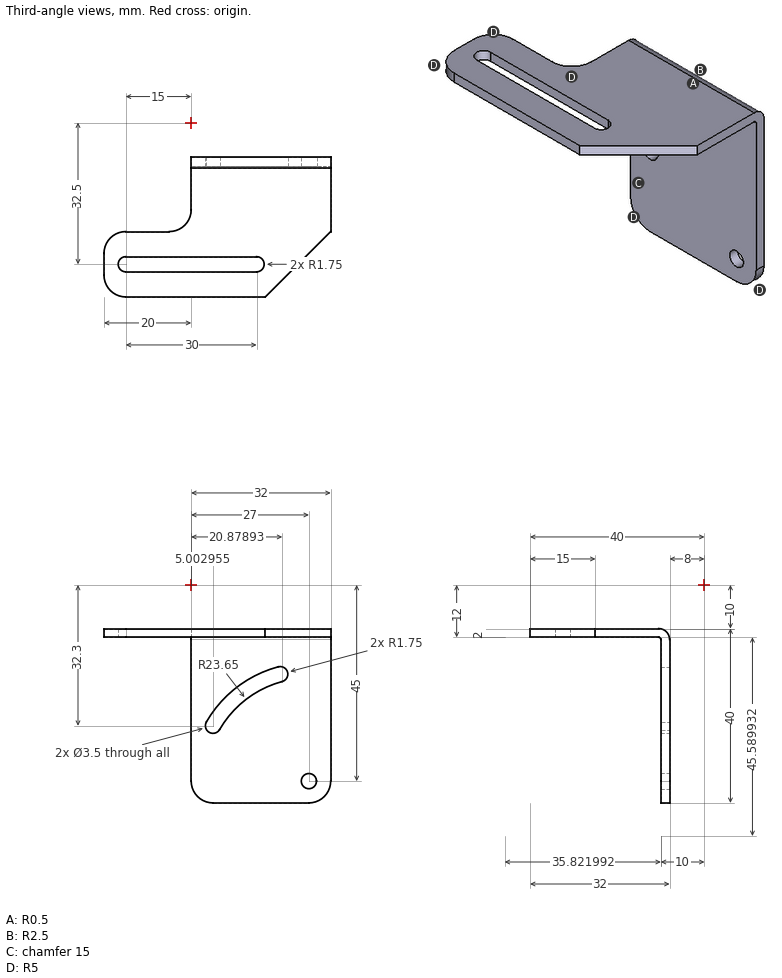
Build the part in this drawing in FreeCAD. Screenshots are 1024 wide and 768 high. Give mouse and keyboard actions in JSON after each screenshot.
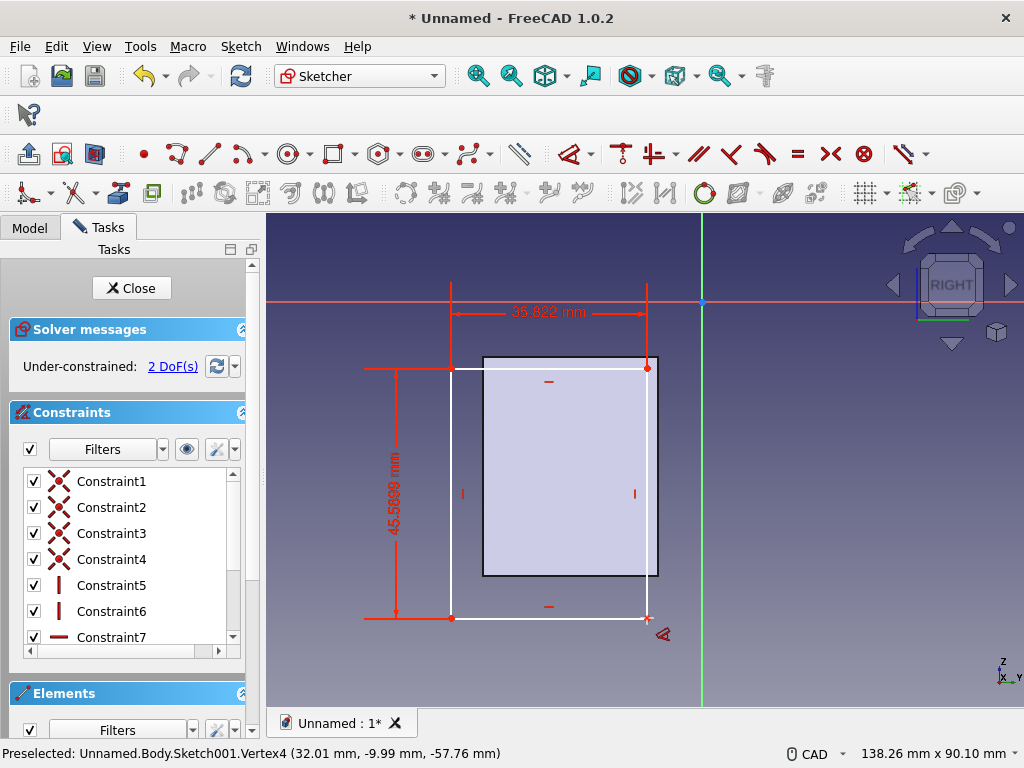
{"action": "left_click", "coordinate": [451, 369]}
{"action": "left_click", "coordinate": [736, 336]}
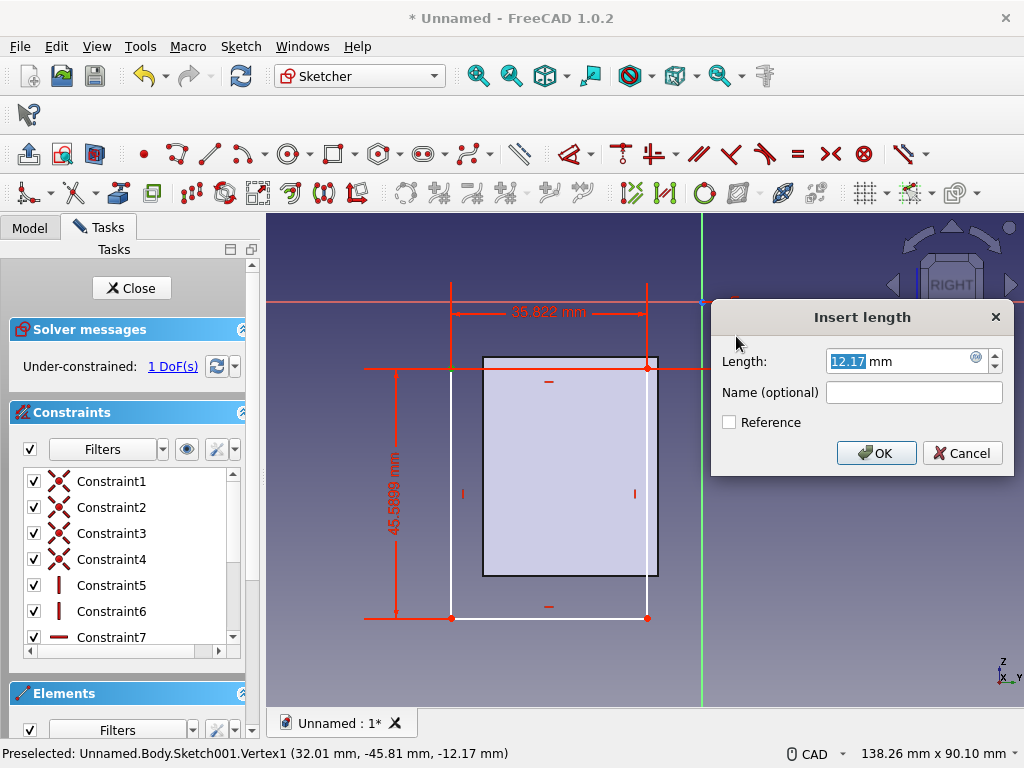
{"action": "type", "text": "12"}
{"action": "key", "text": "Return"}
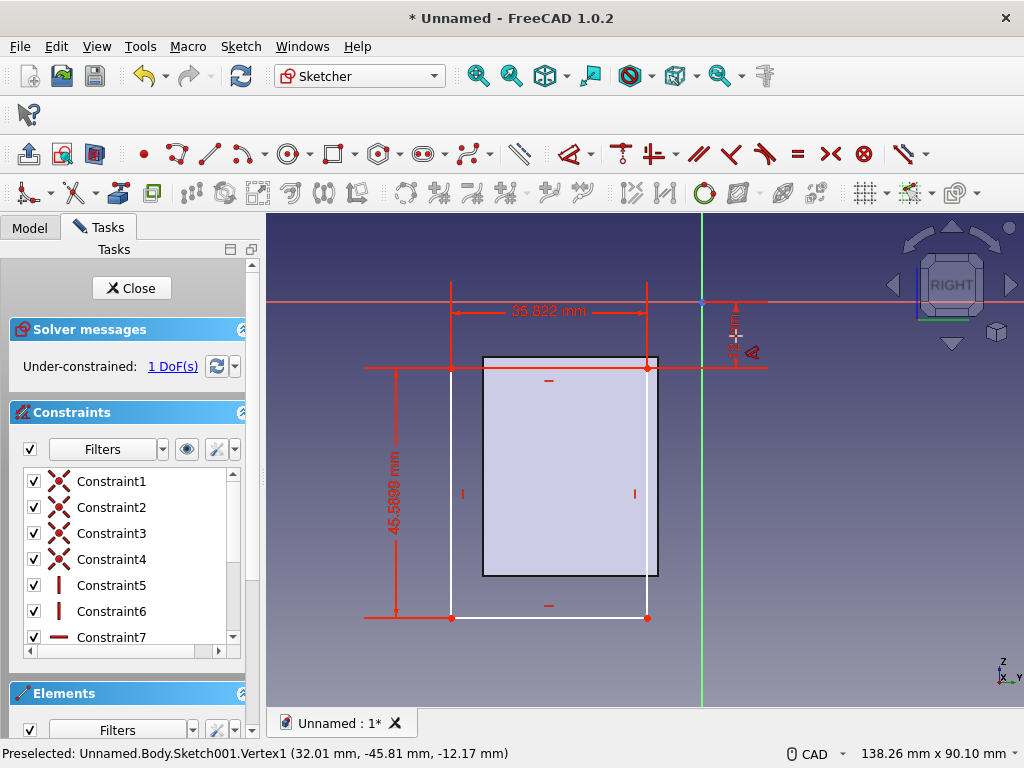
{"action": "left_click", "coordinate": [647, 618]}
{"action": "left_click", "coordinate": [675, 268]}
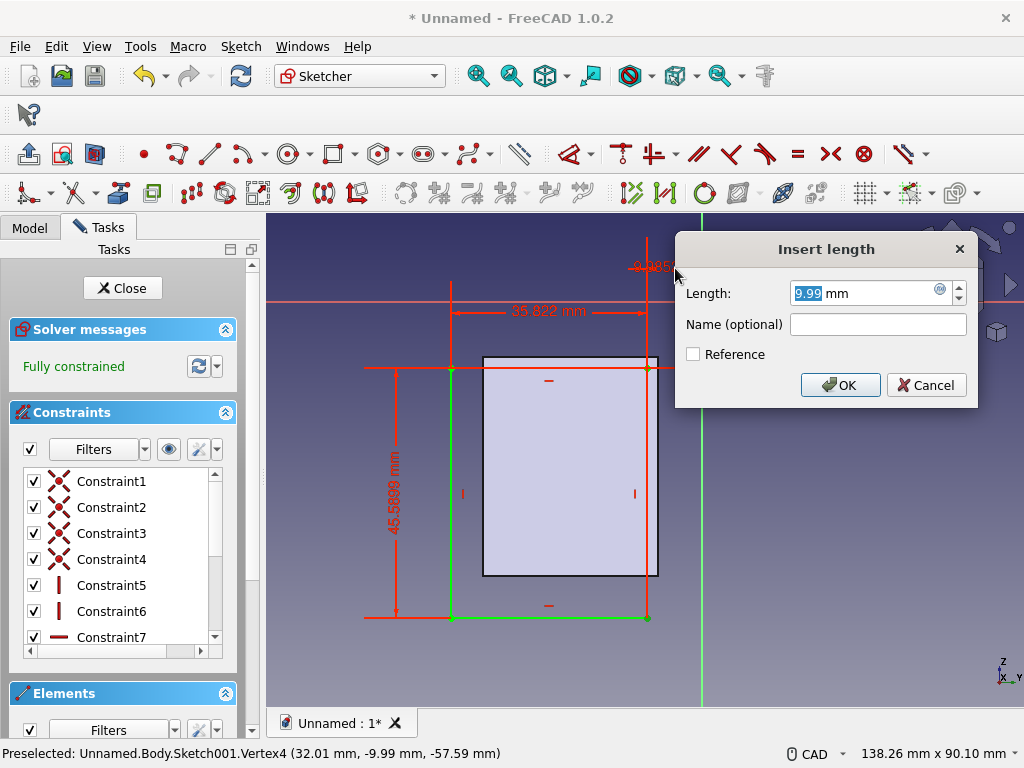
{"action": "type", "text": "10"}
{"action": "key", "text": "Return"}
{"action": "key", "text": "Escape"}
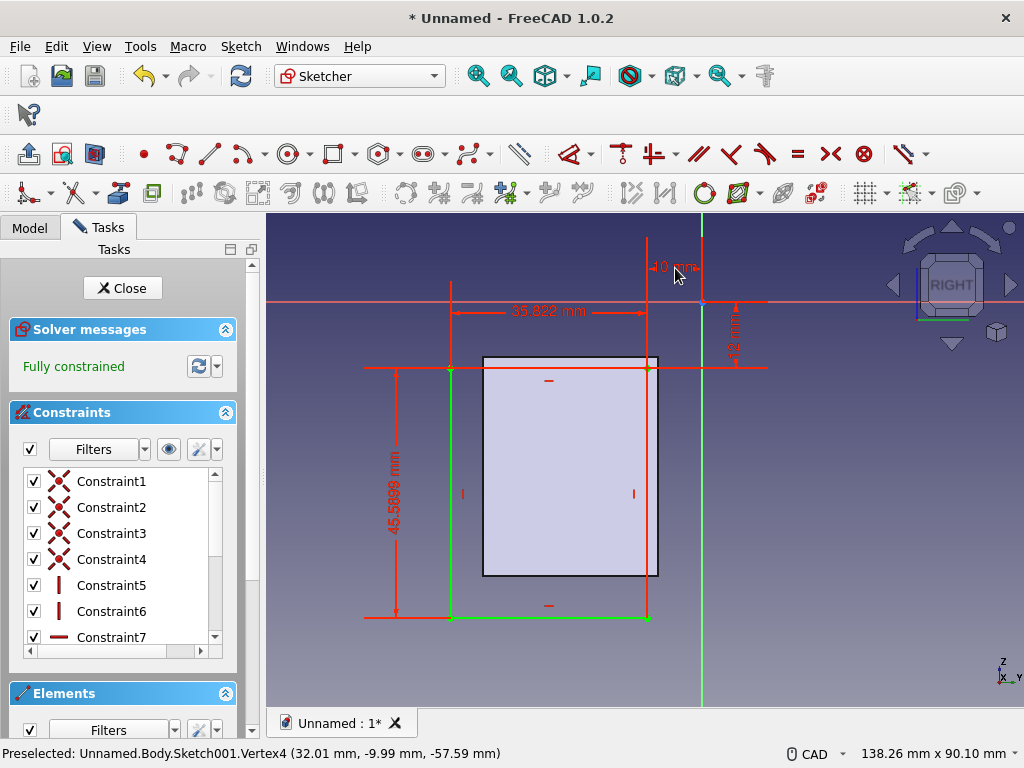
{"action": "left_click", "coordinate": [123, 288]}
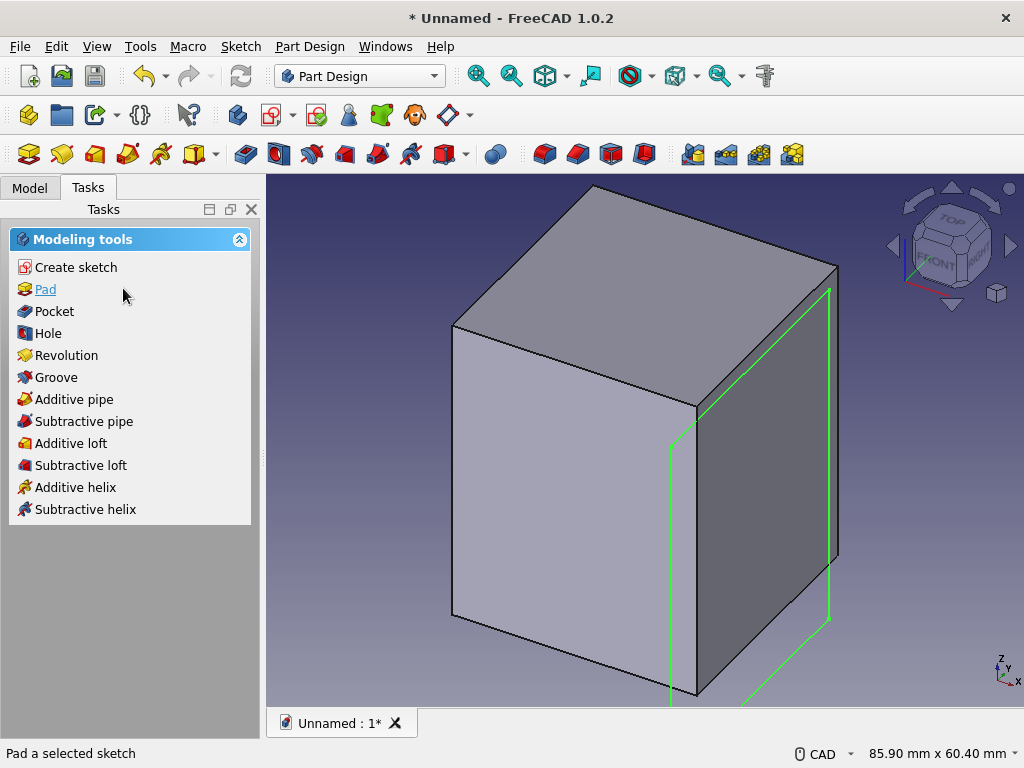
{"action": "left_click", "coordinate": [246, 154]}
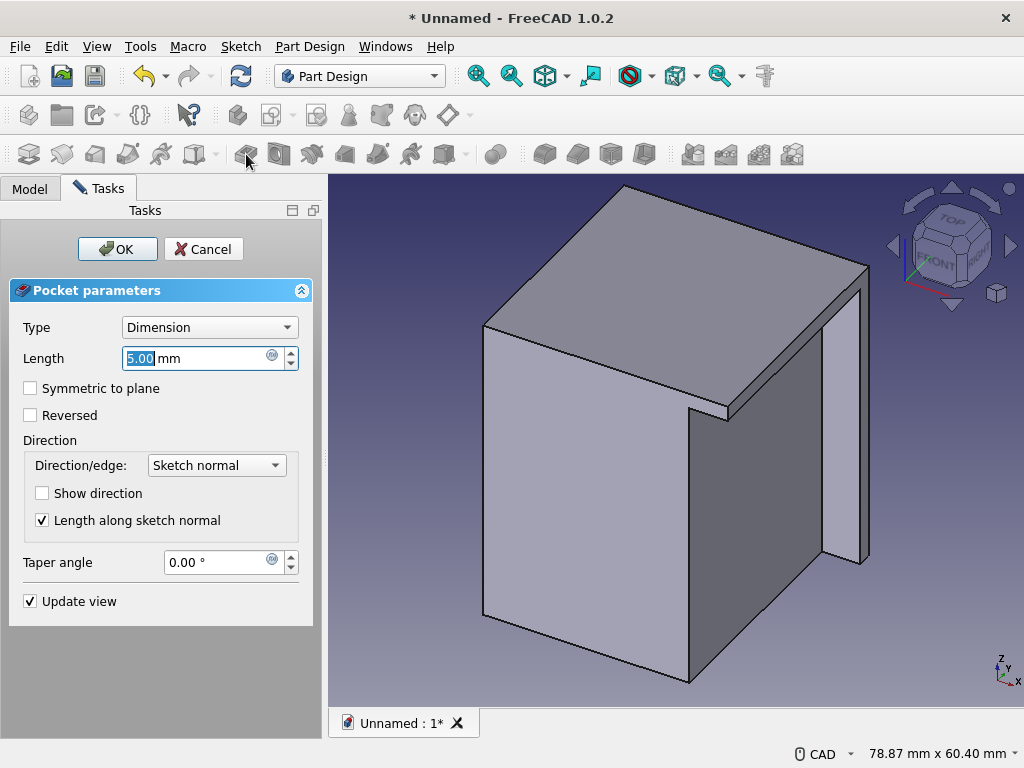
{"action": "left_click", "coordinate": [210, 328]}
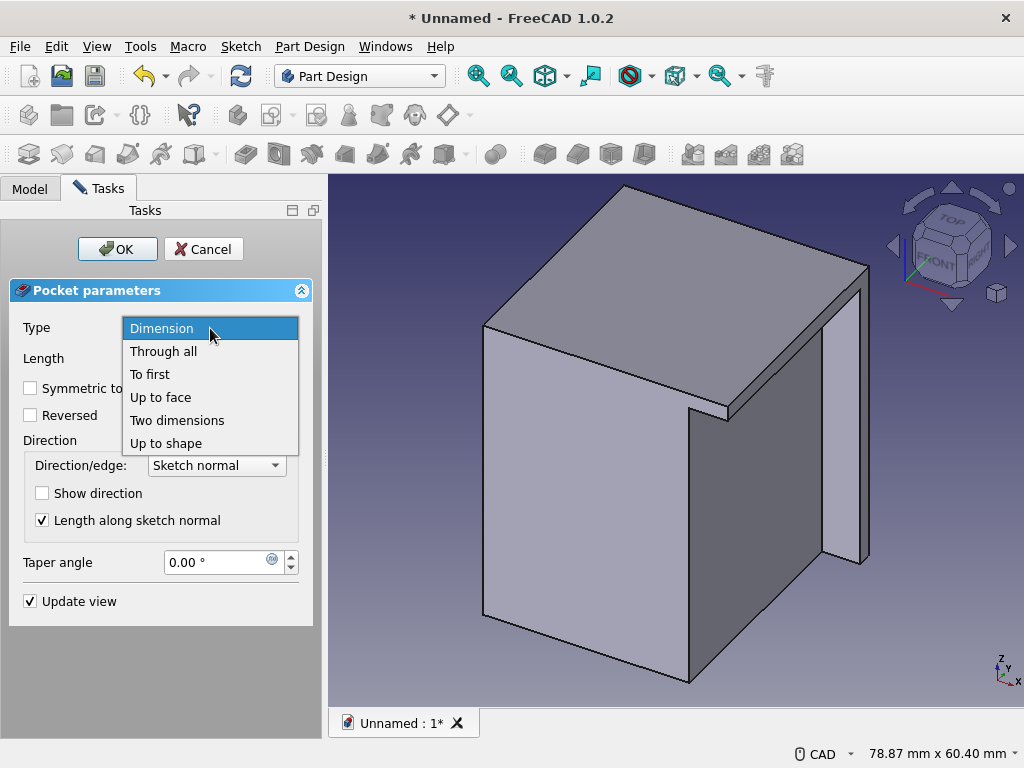
{"action": "left_click", "coordinate": [208, 352]}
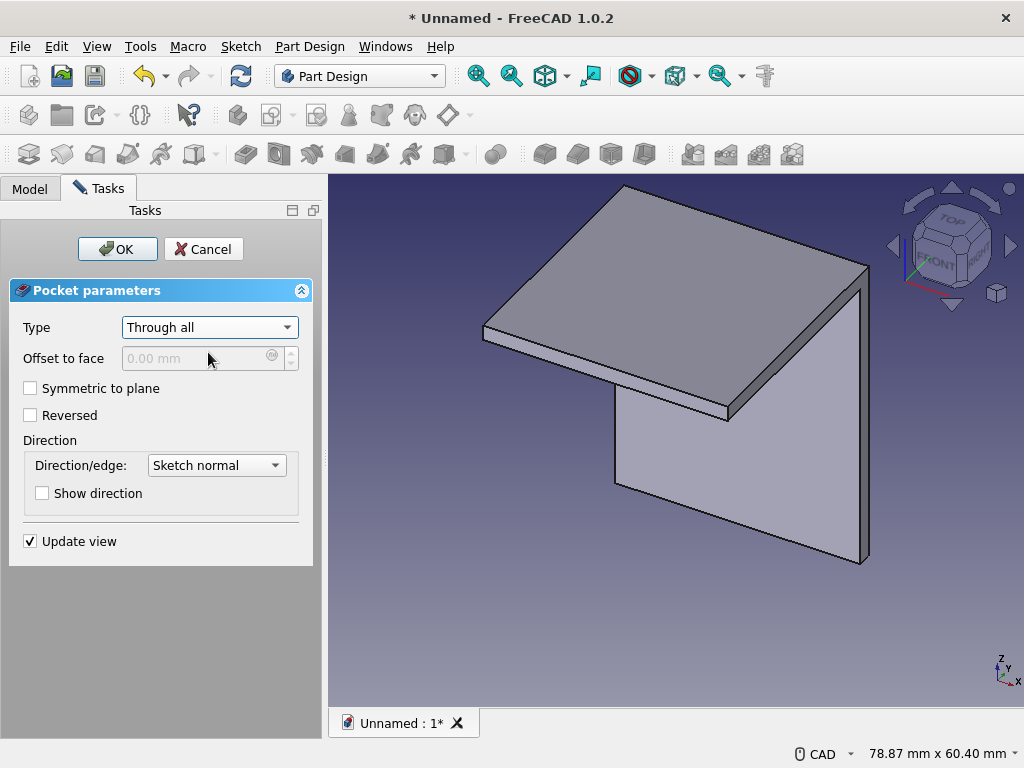
{"action": "left_click", "coordinate": [118, 249]}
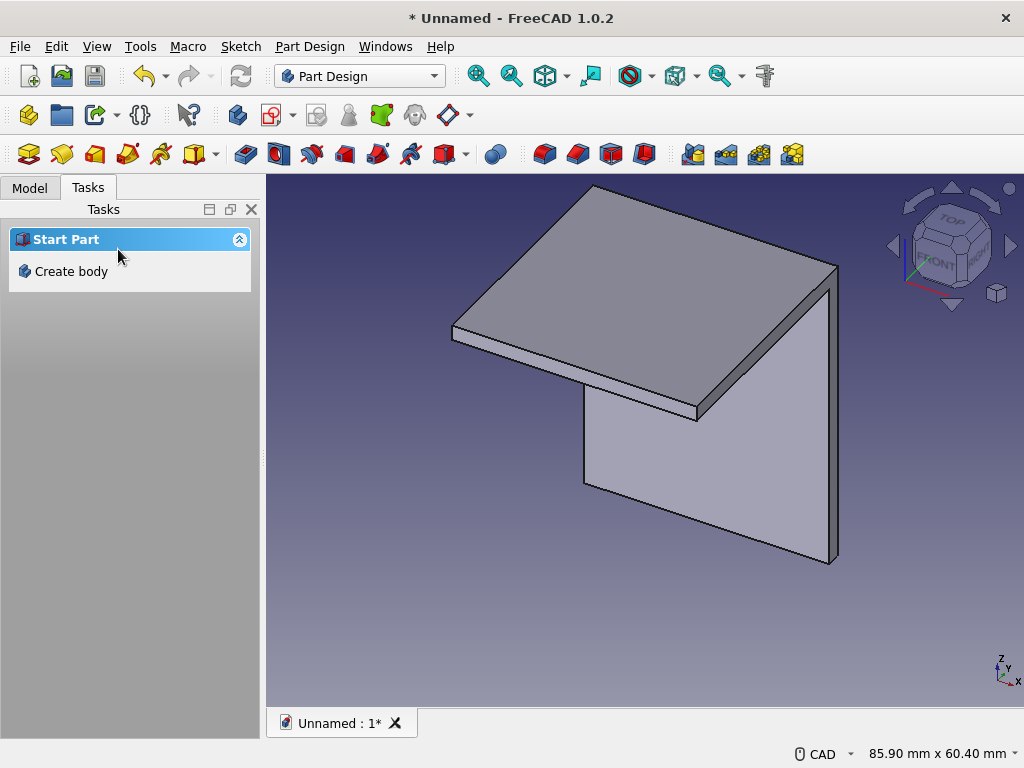
{"action": "left_click", "coordinate": [707, 425]}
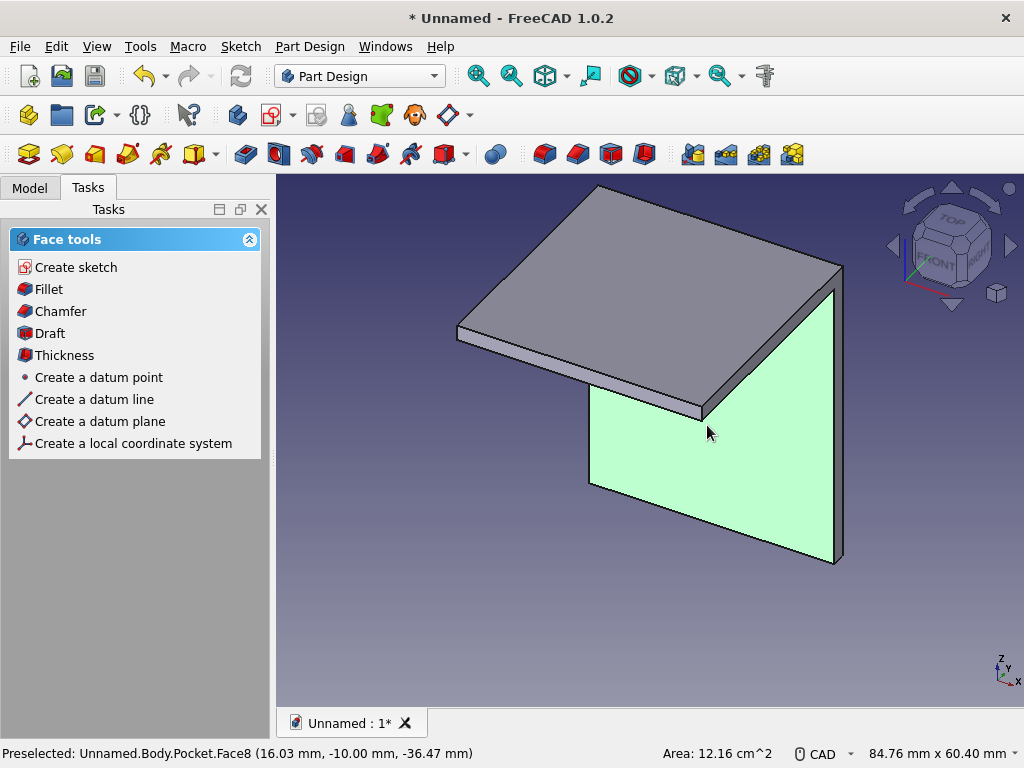
{"action": "left_click", "coordinate": [270, 116]}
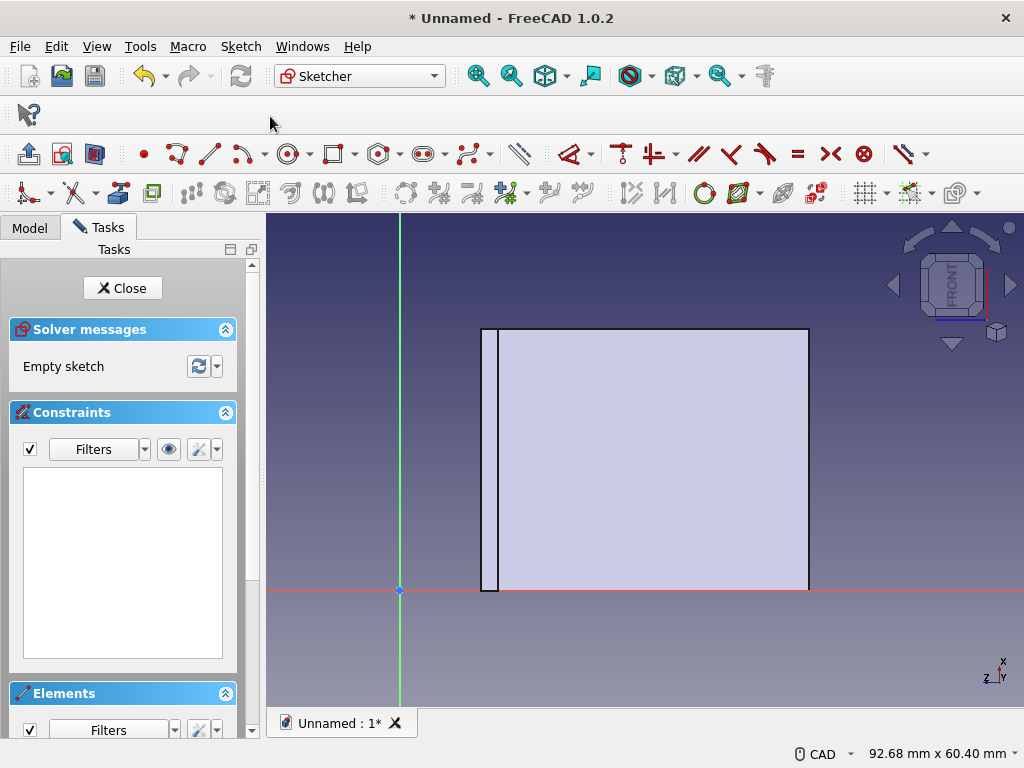
{"action": "key", "text": "g c"}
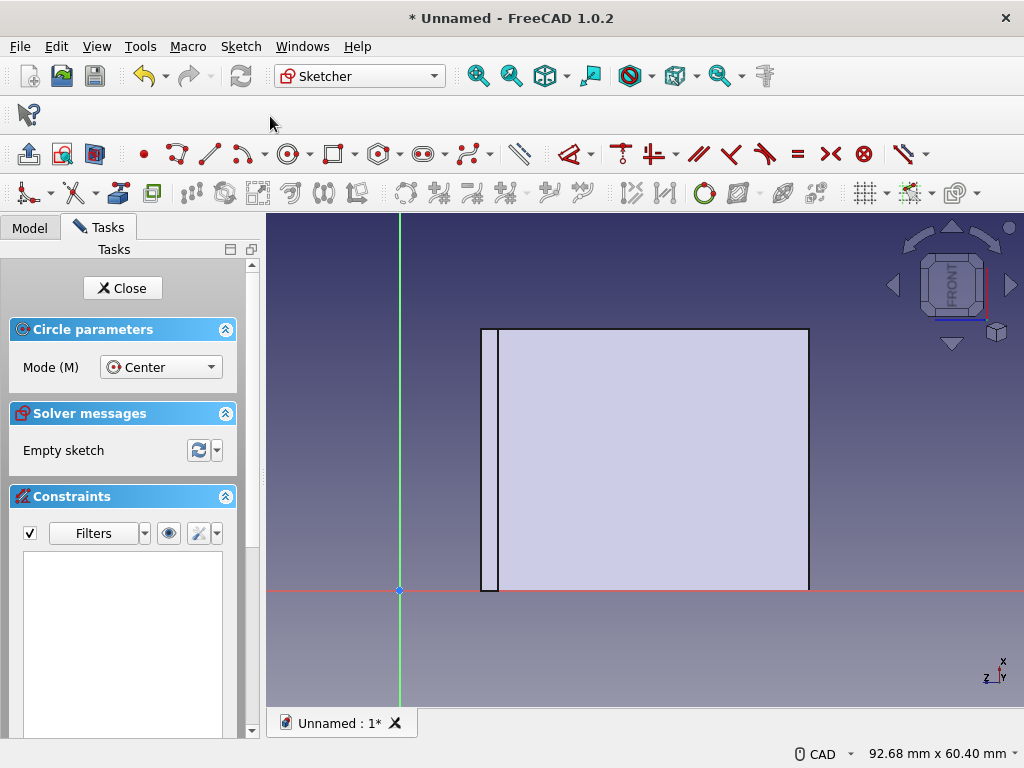
{"action": "scroll", "coordinate": [664, 550], "scroll_direction": "up", "scroll_amount": 3}